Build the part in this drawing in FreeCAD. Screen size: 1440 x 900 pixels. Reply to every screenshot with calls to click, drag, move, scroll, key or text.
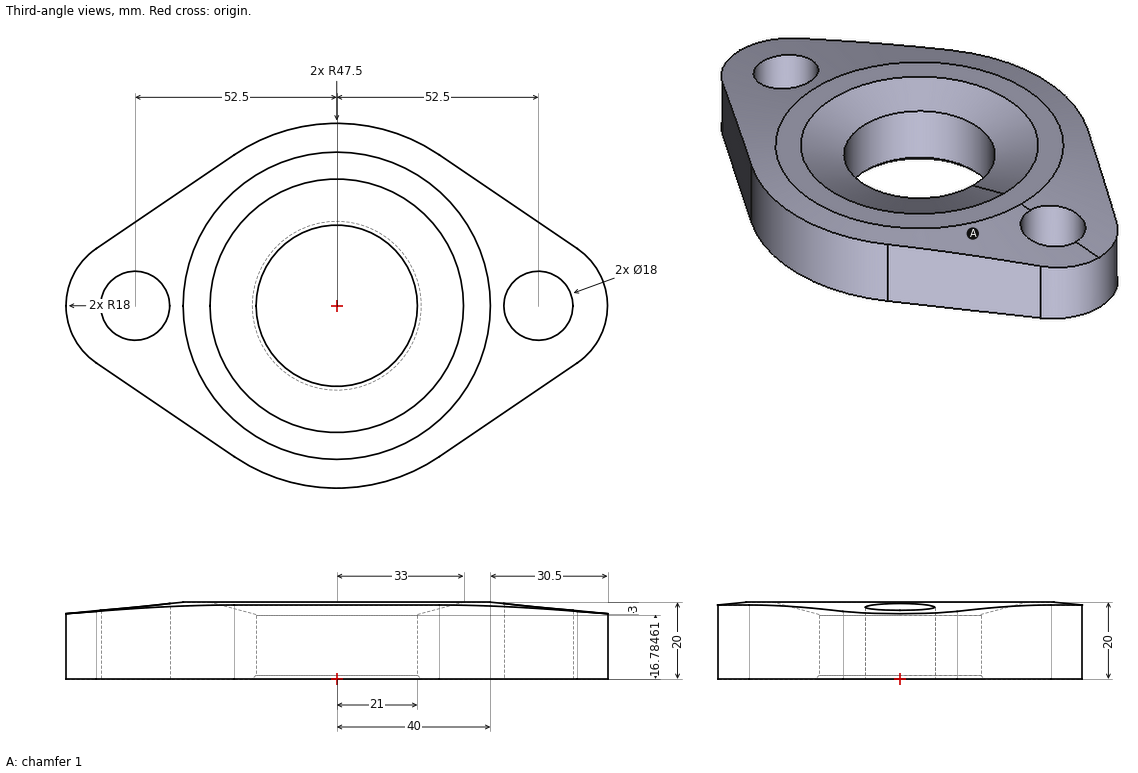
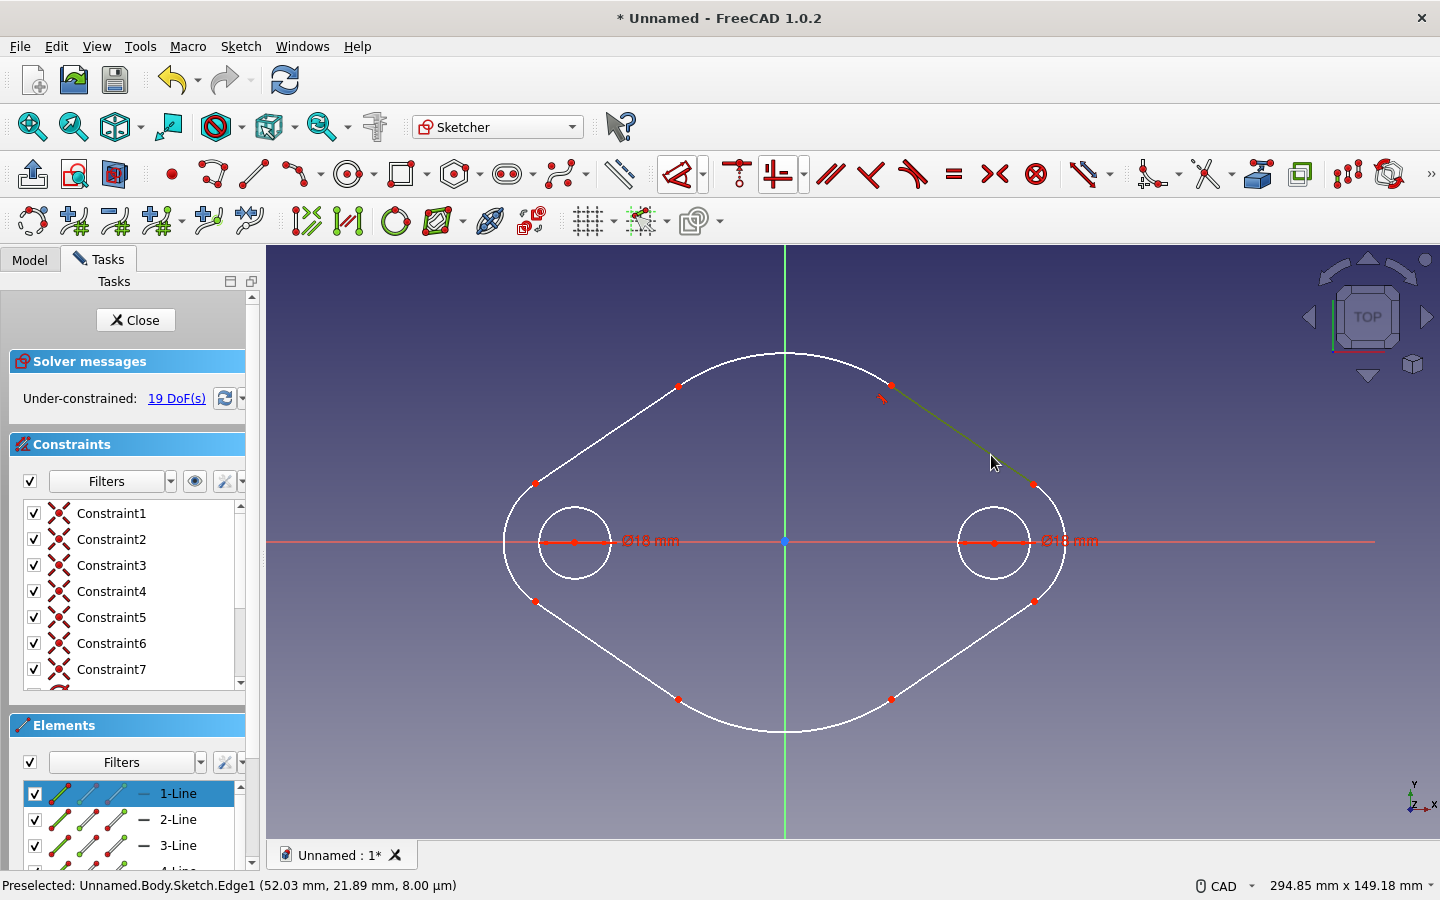
click(1060, 570)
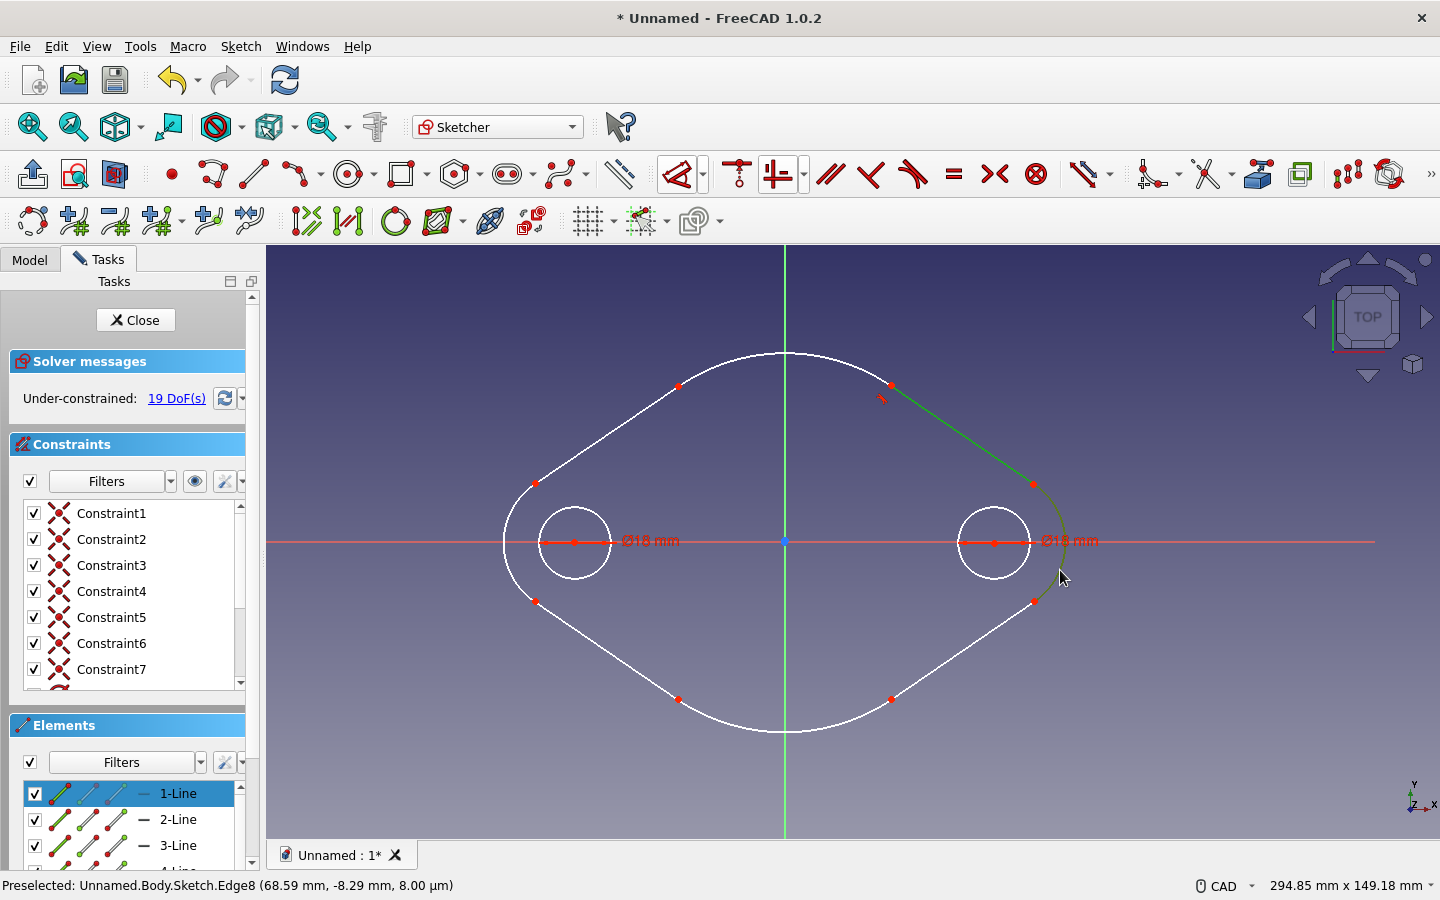
key(t)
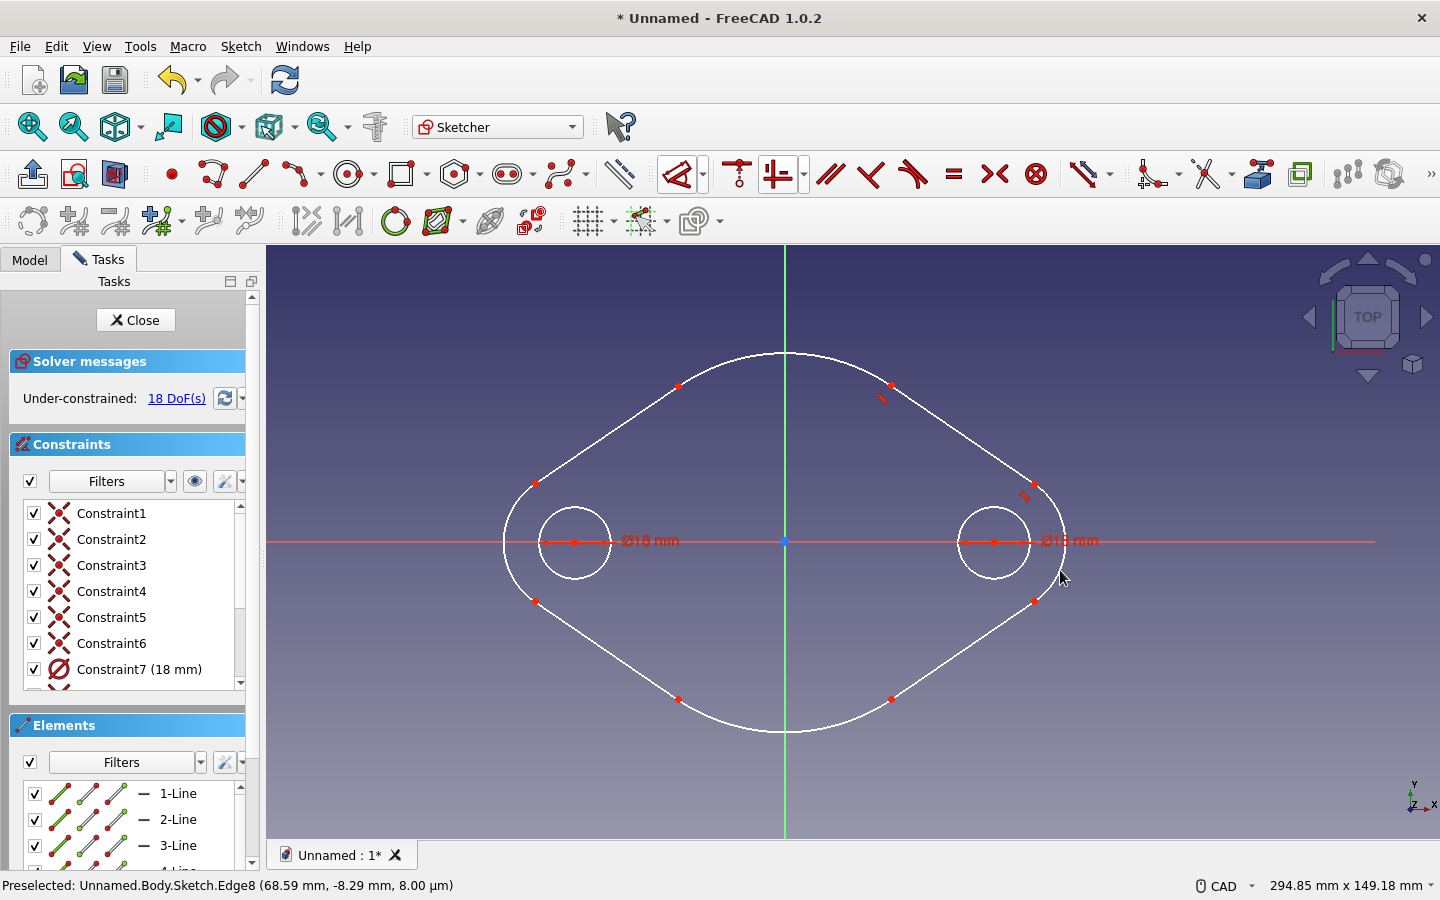
click(635, 416)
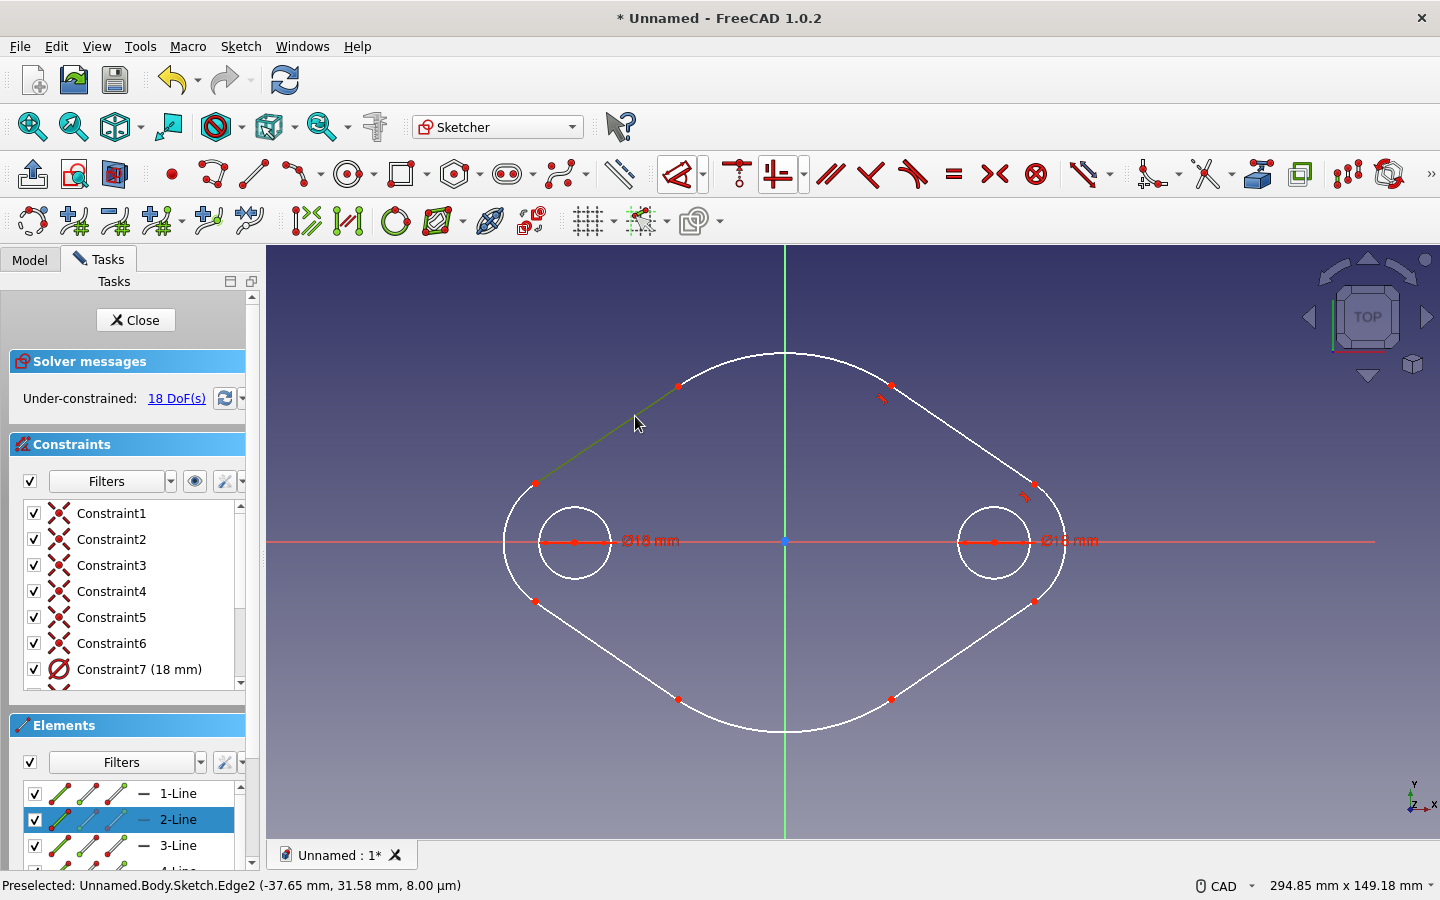
click(829, 358)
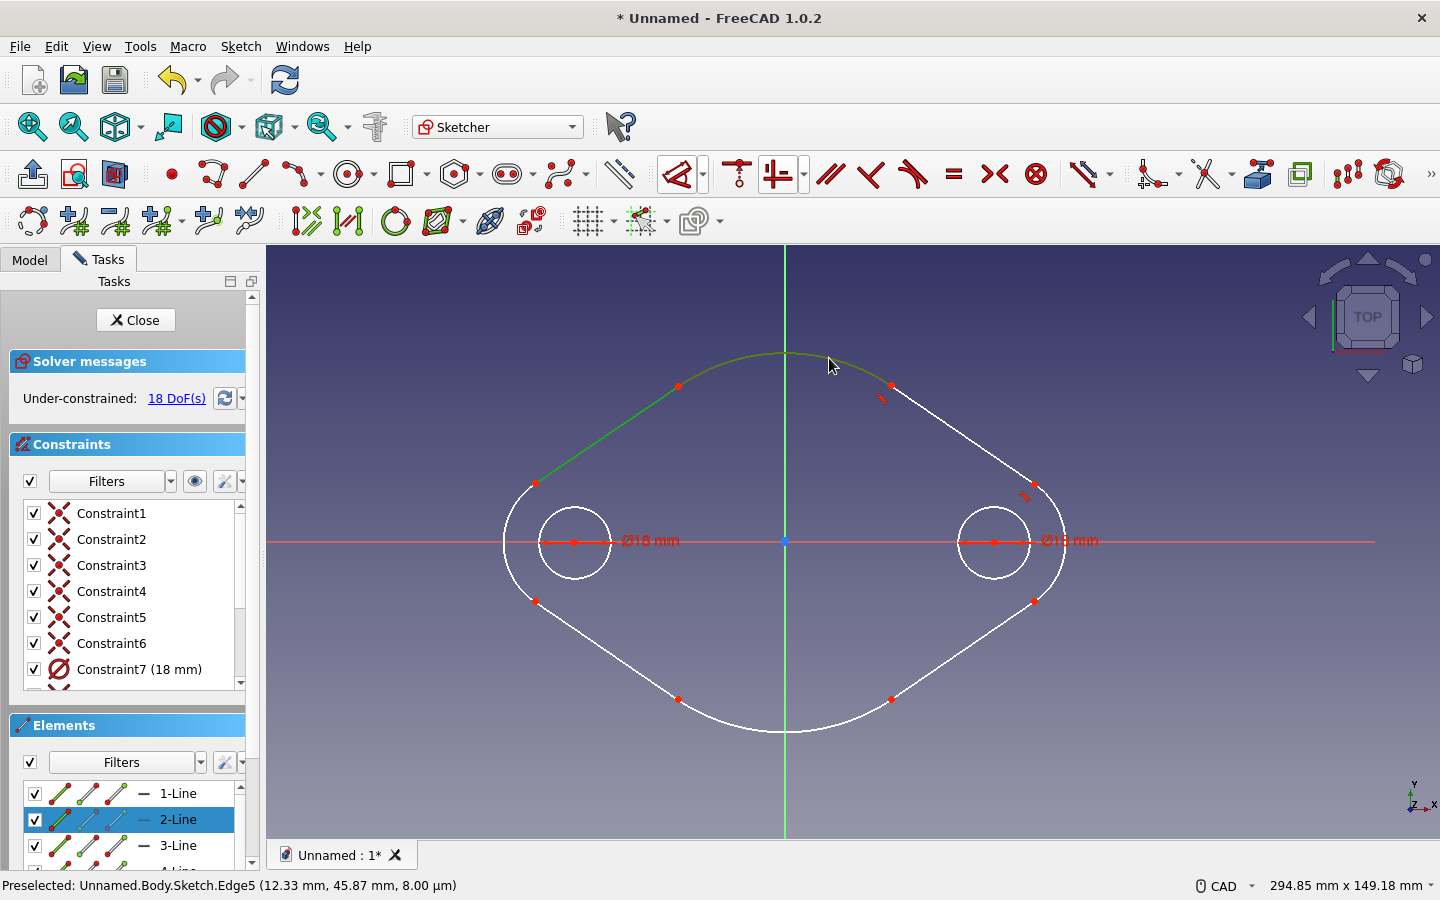
click(913, 174)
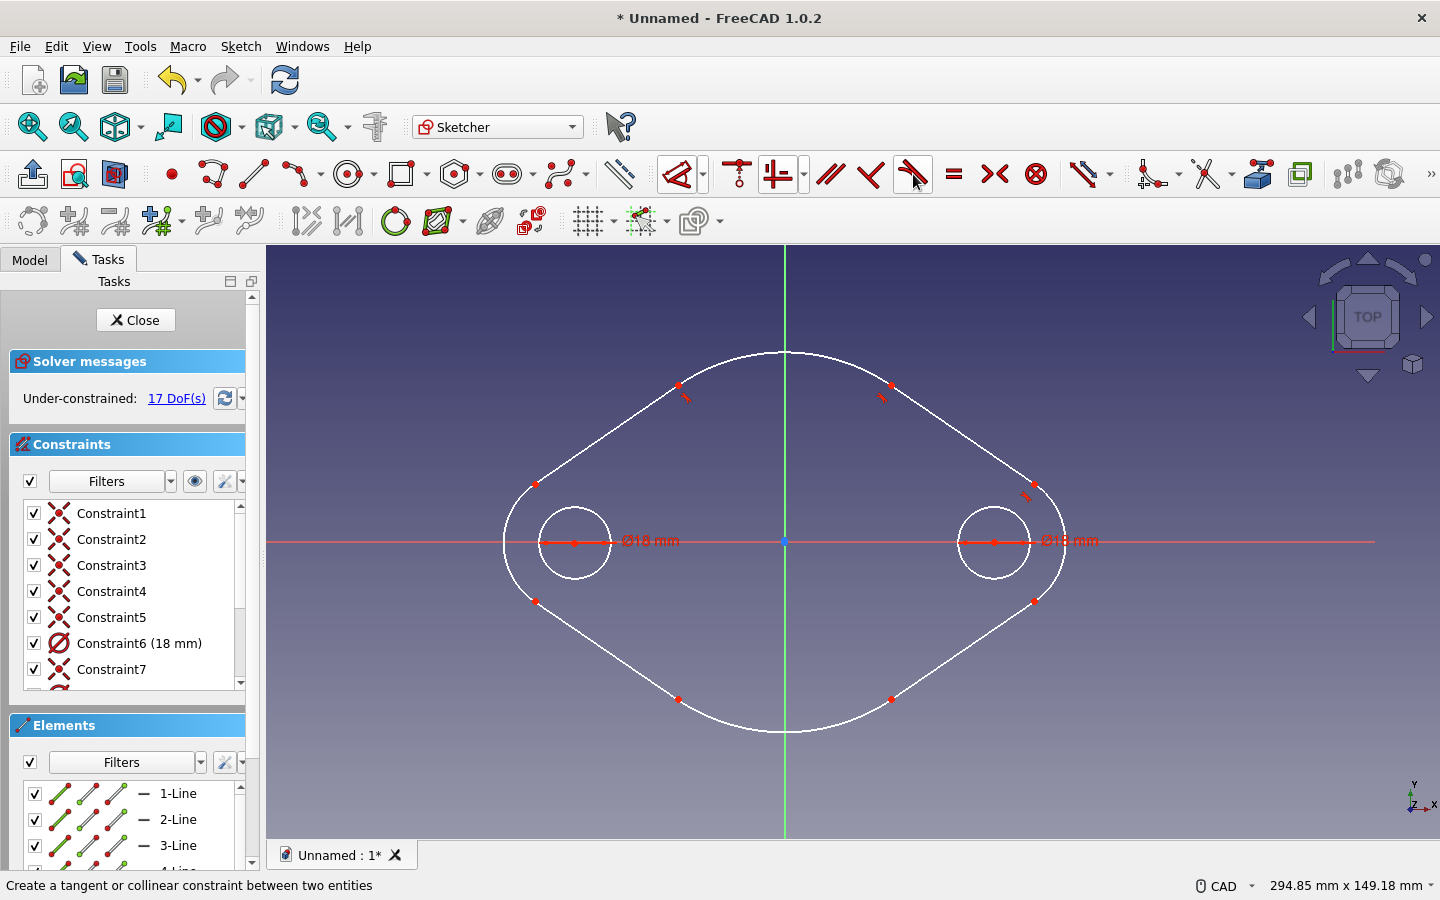
click(635, 415)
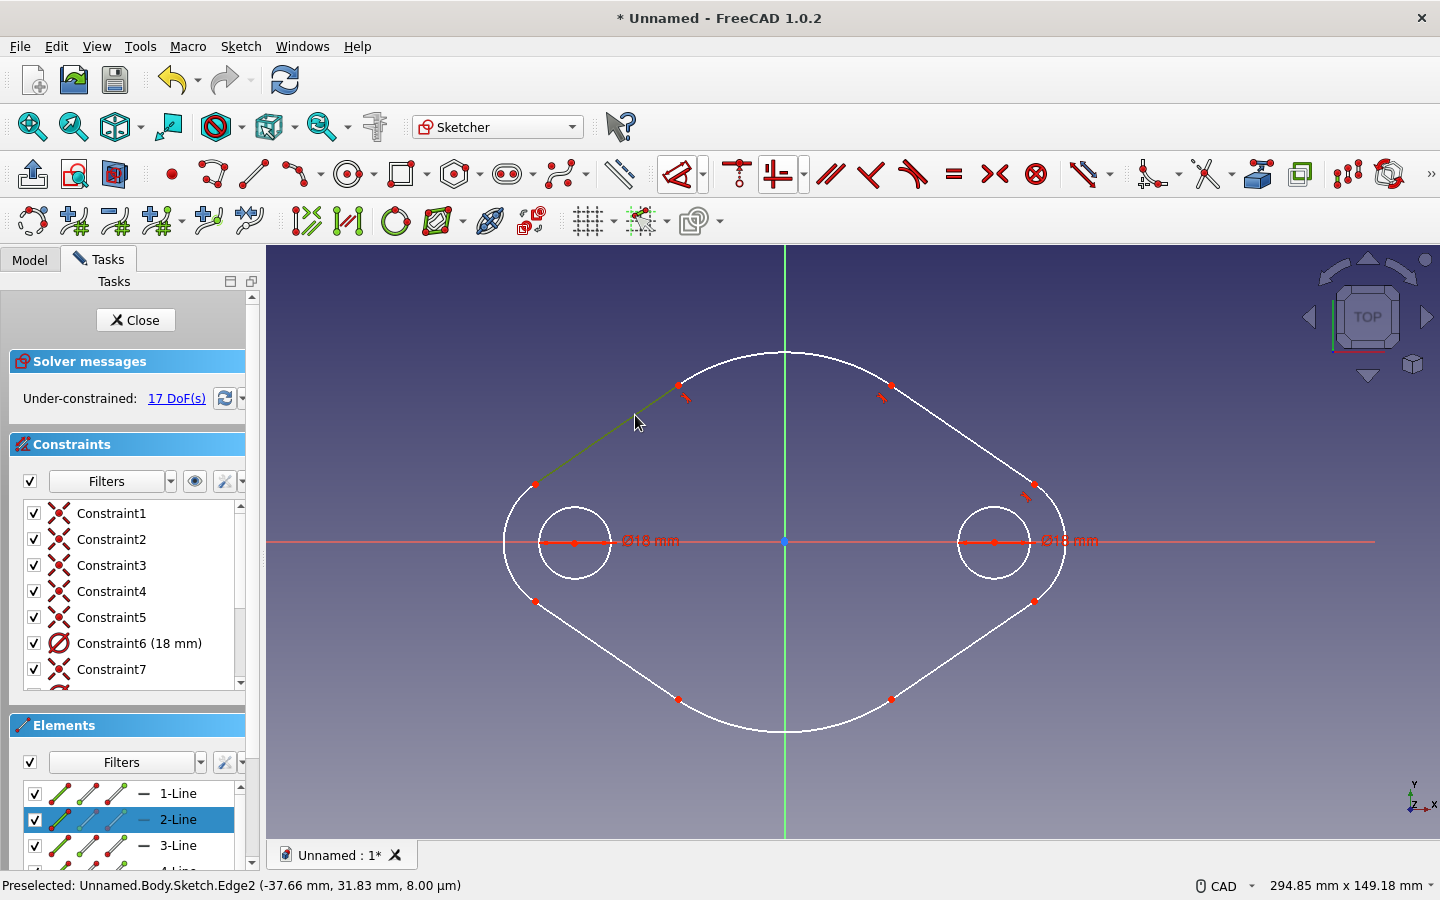
click(509, 516)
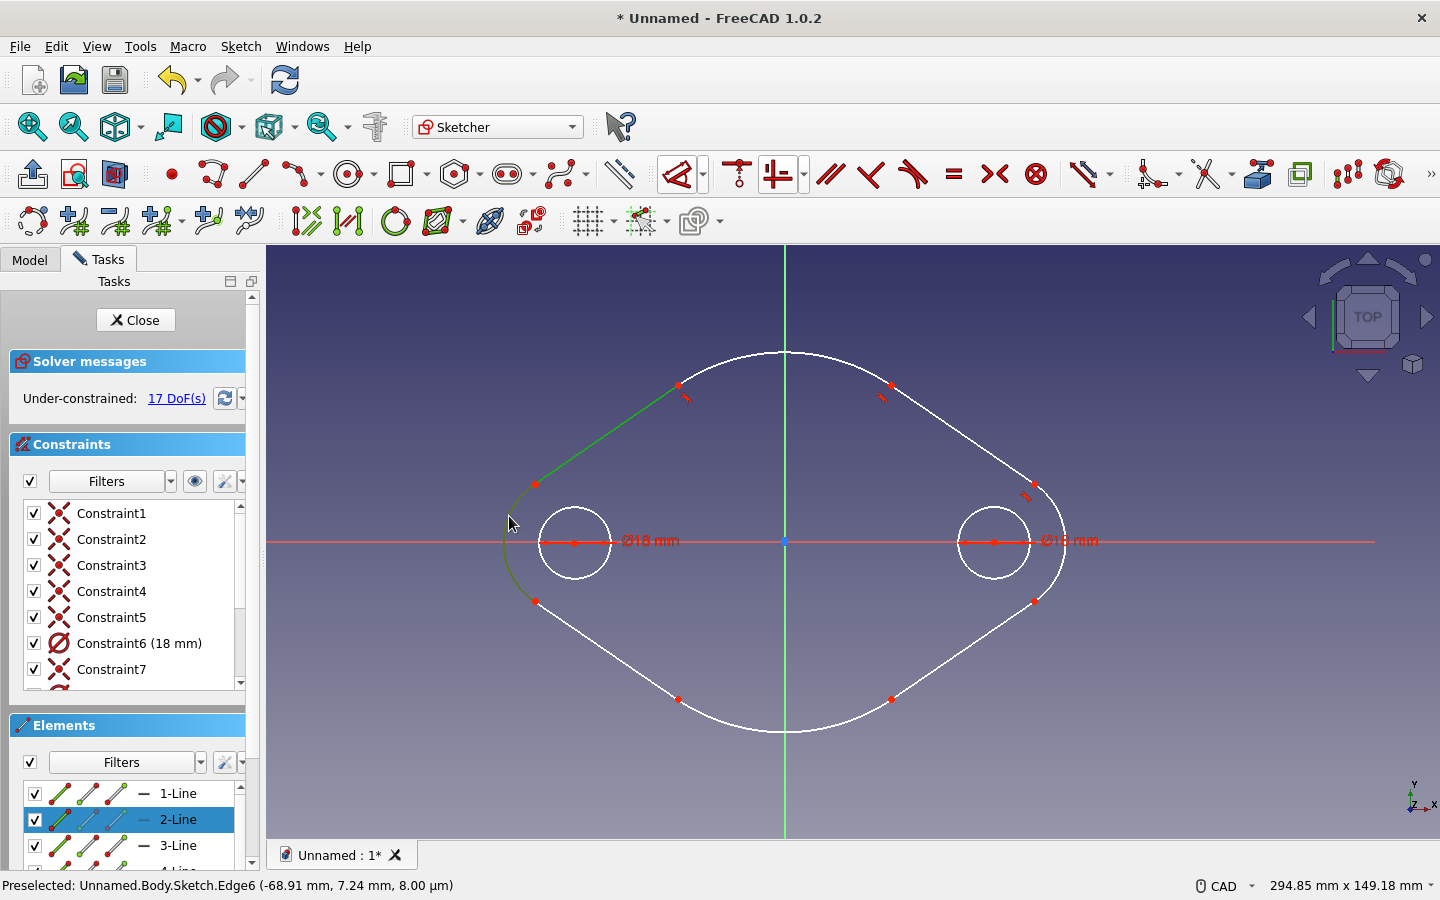
key(t)